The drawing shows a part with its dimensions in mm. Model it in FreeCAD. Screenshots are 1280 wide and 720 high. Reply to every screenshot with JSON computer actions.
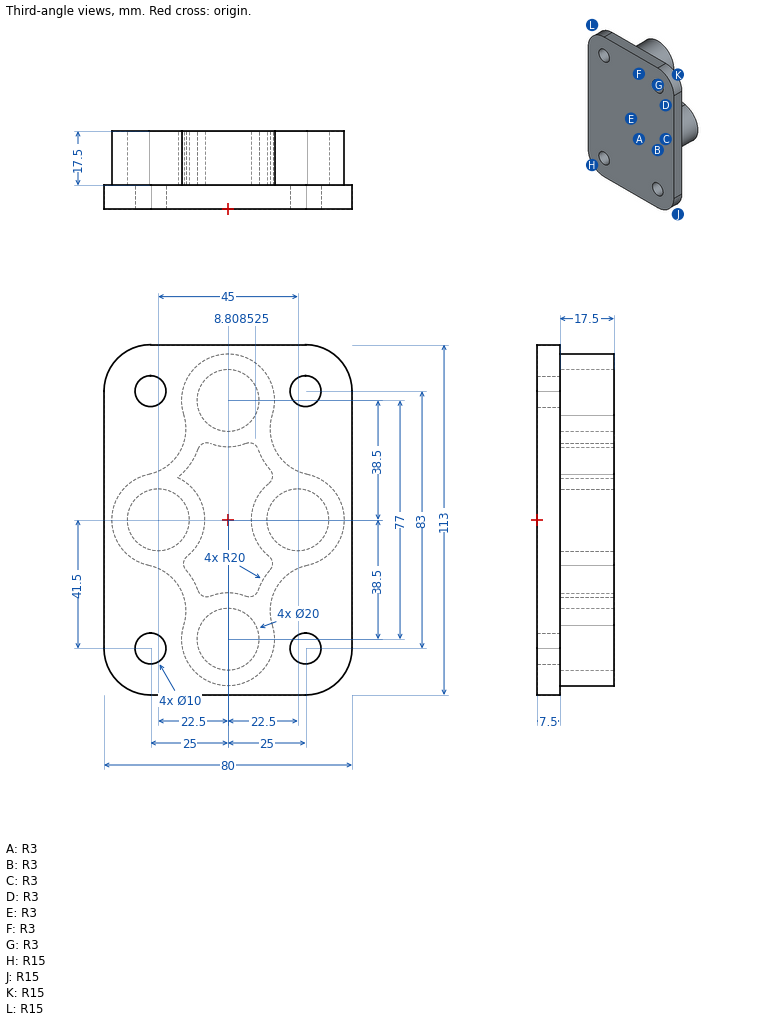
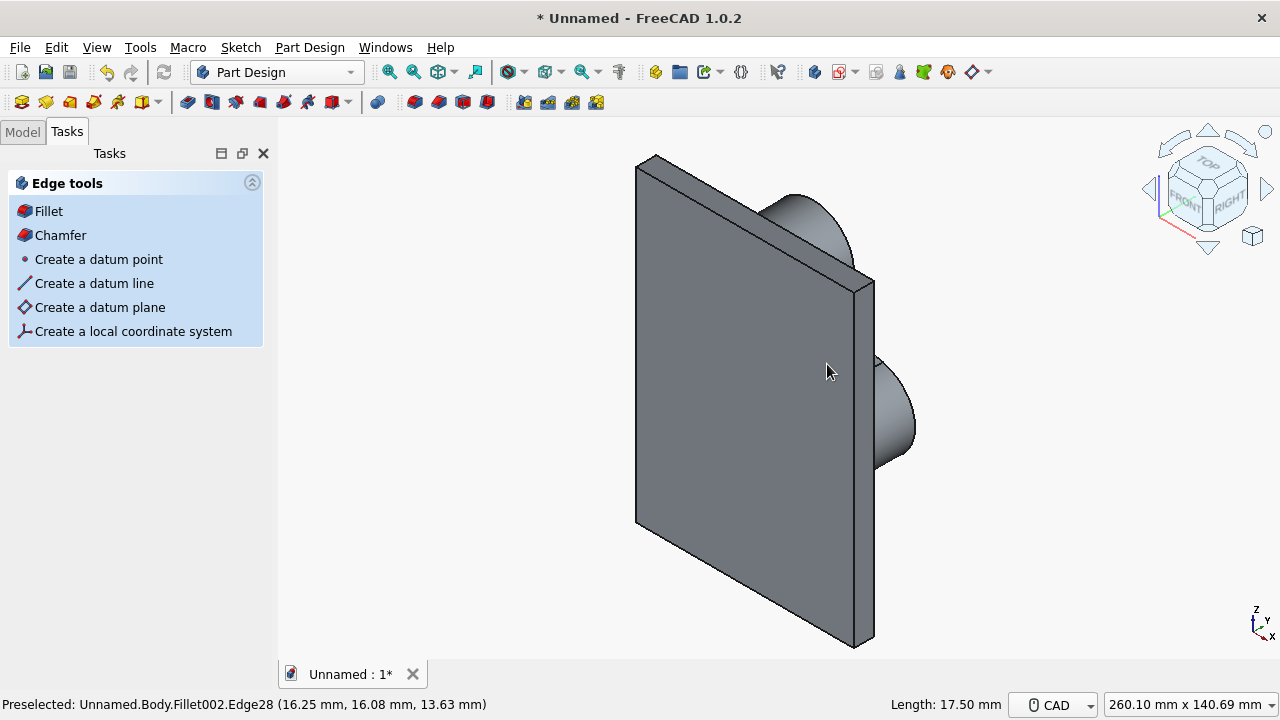
{"action": "left_click", "coordinate": [416, 102]}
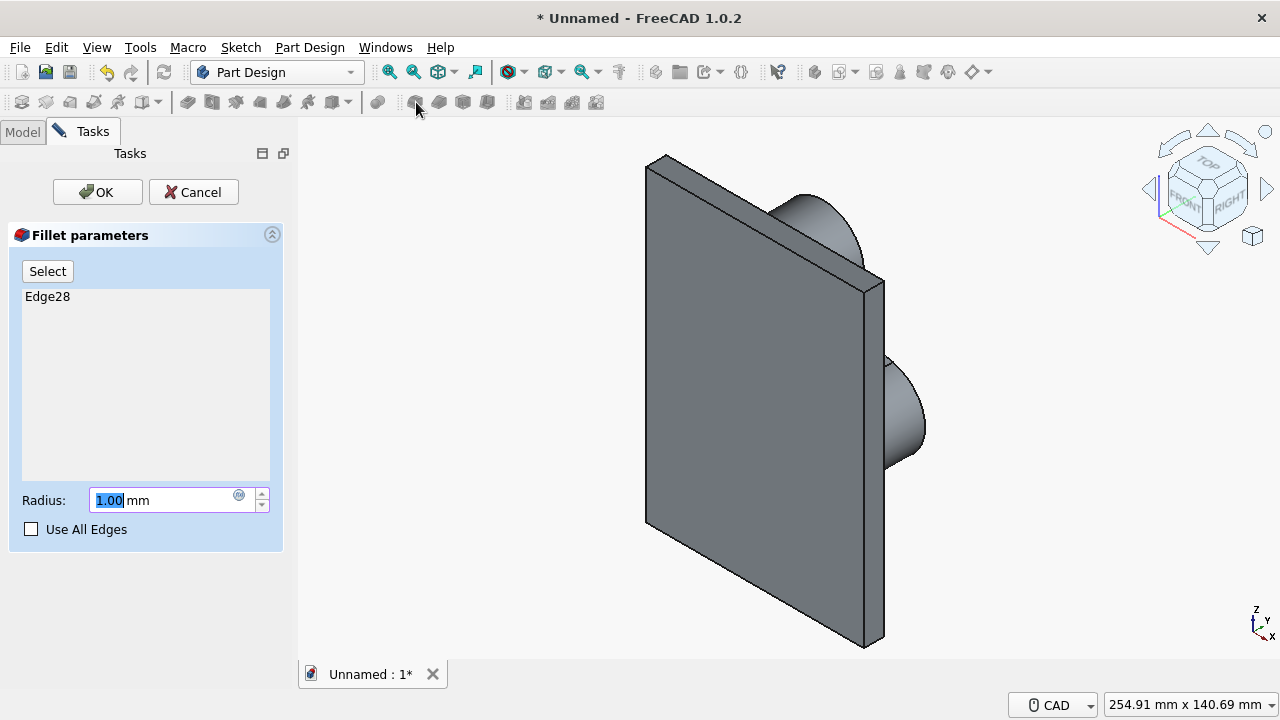
{"action": "type", "text": "3"}
{"action": "key", "text": "Tab"}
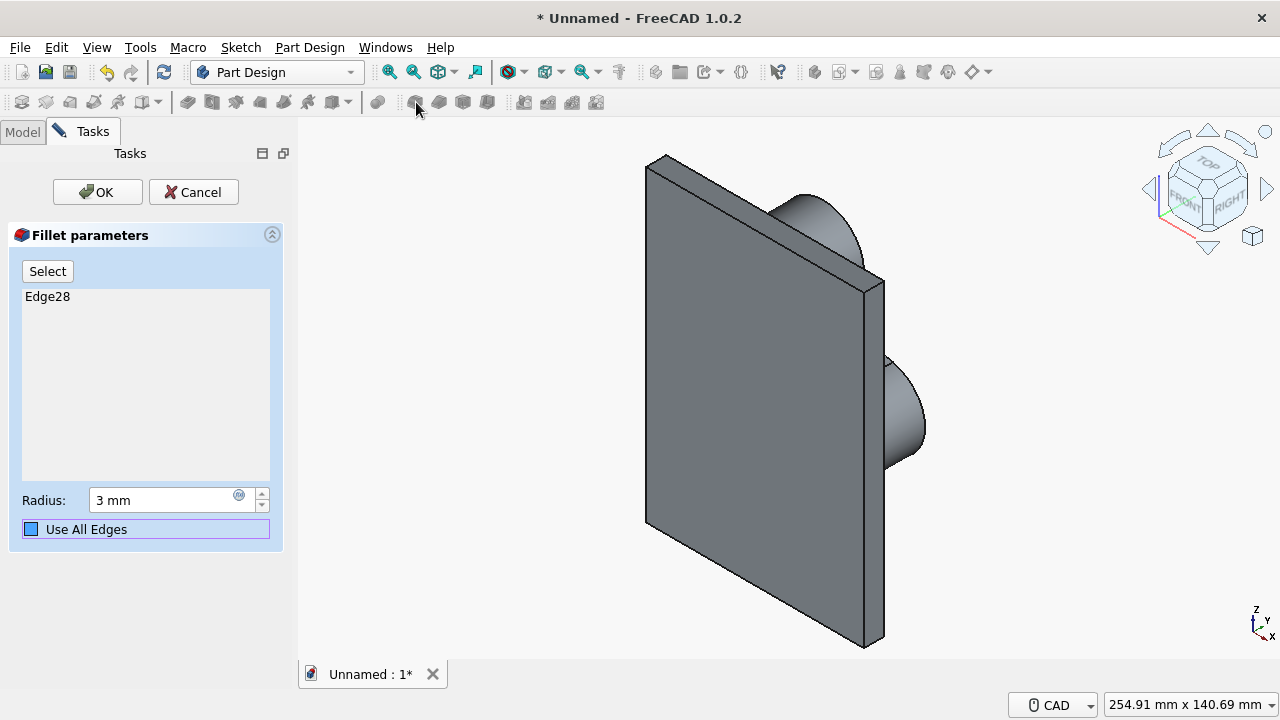
{"action": "left_click", "coordinate": [98, 192]}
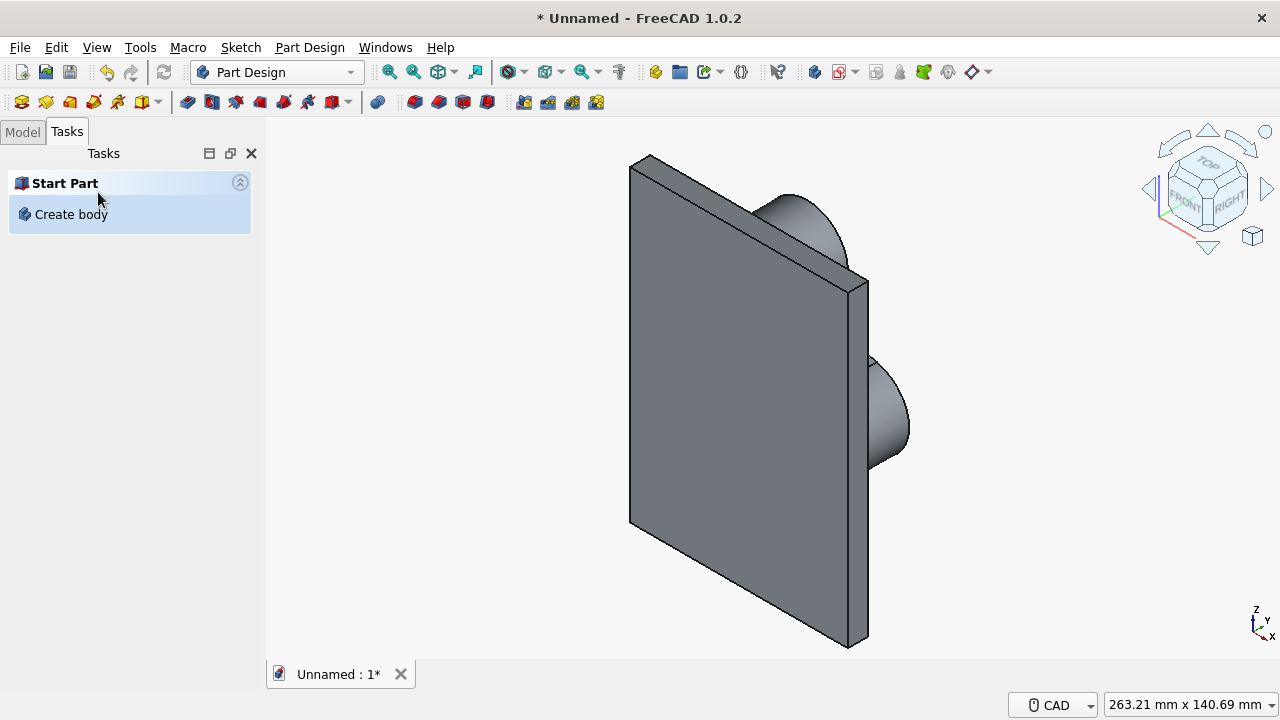
{"action": "key", "text": "2"}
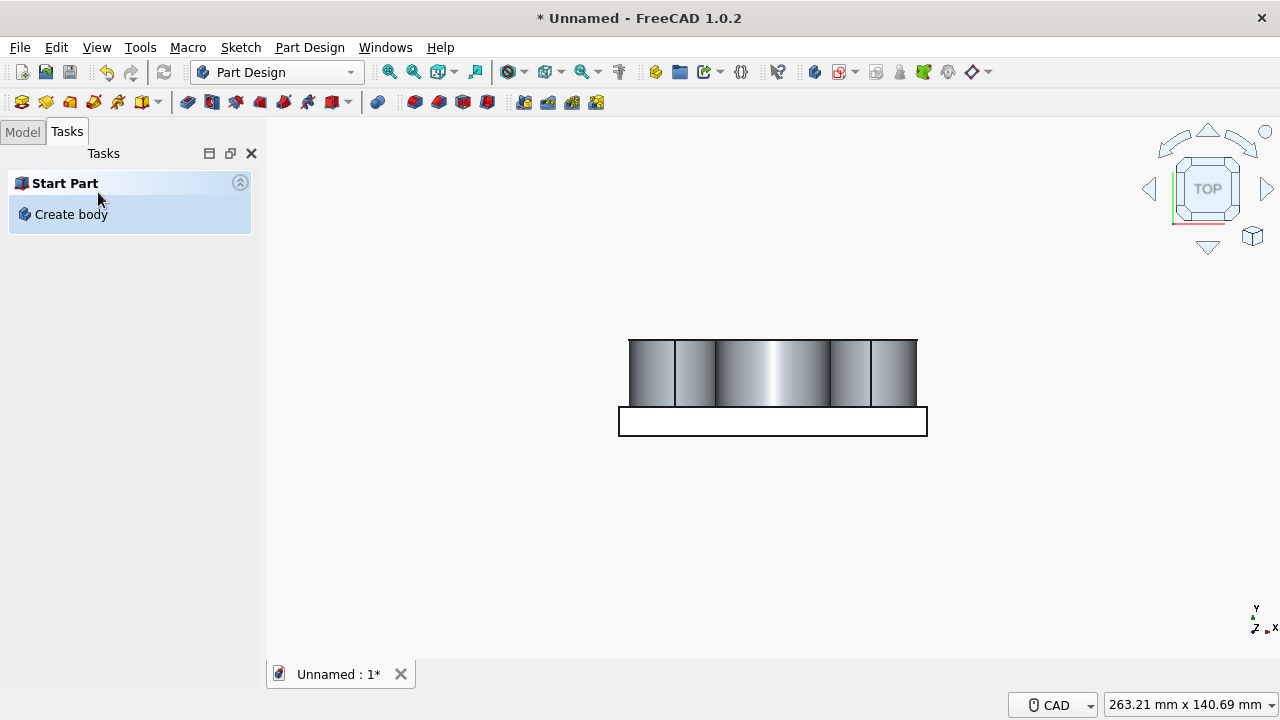
{"action": "key", "text": "v f"}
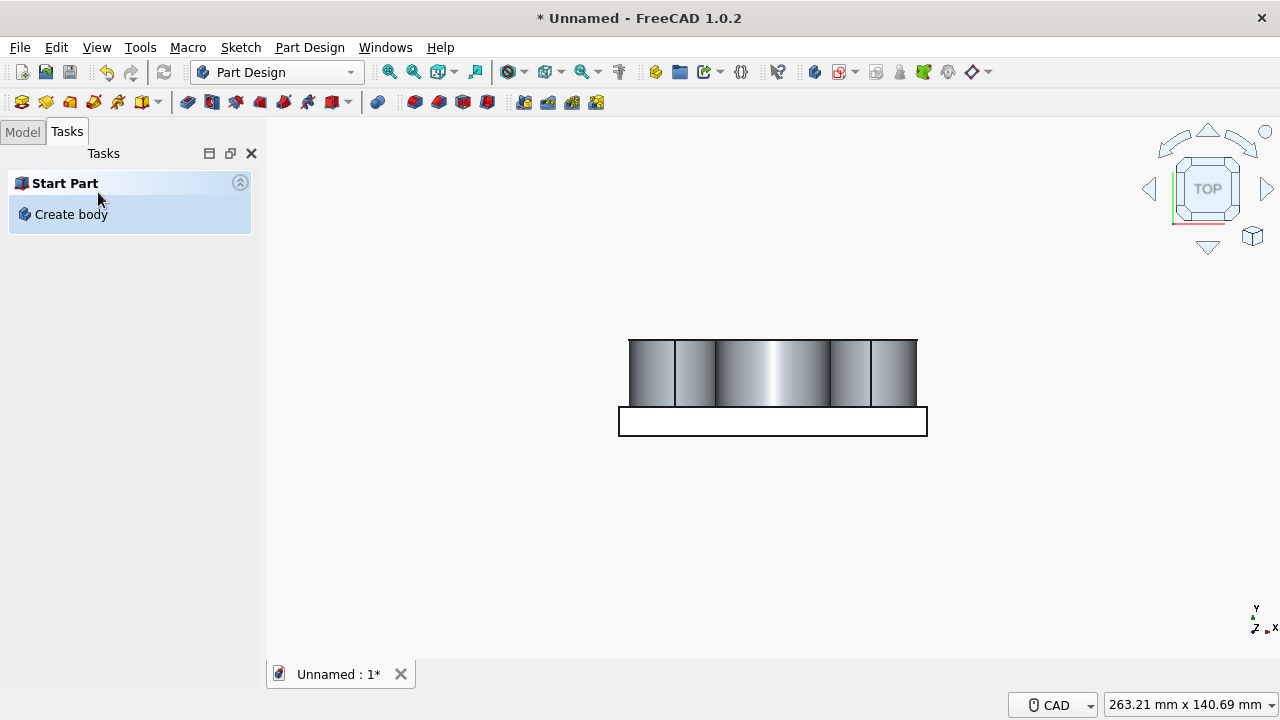
{"action": "key", "text": "0"}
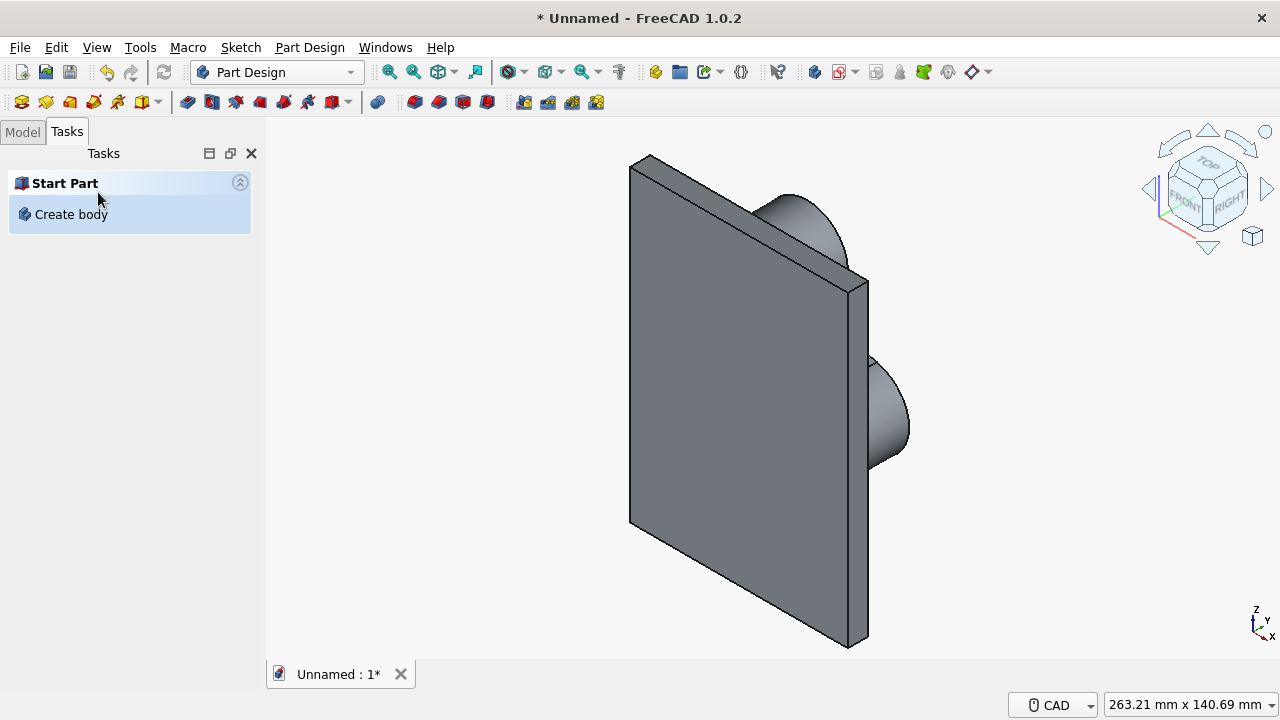
{"action": "key", "text": "1"}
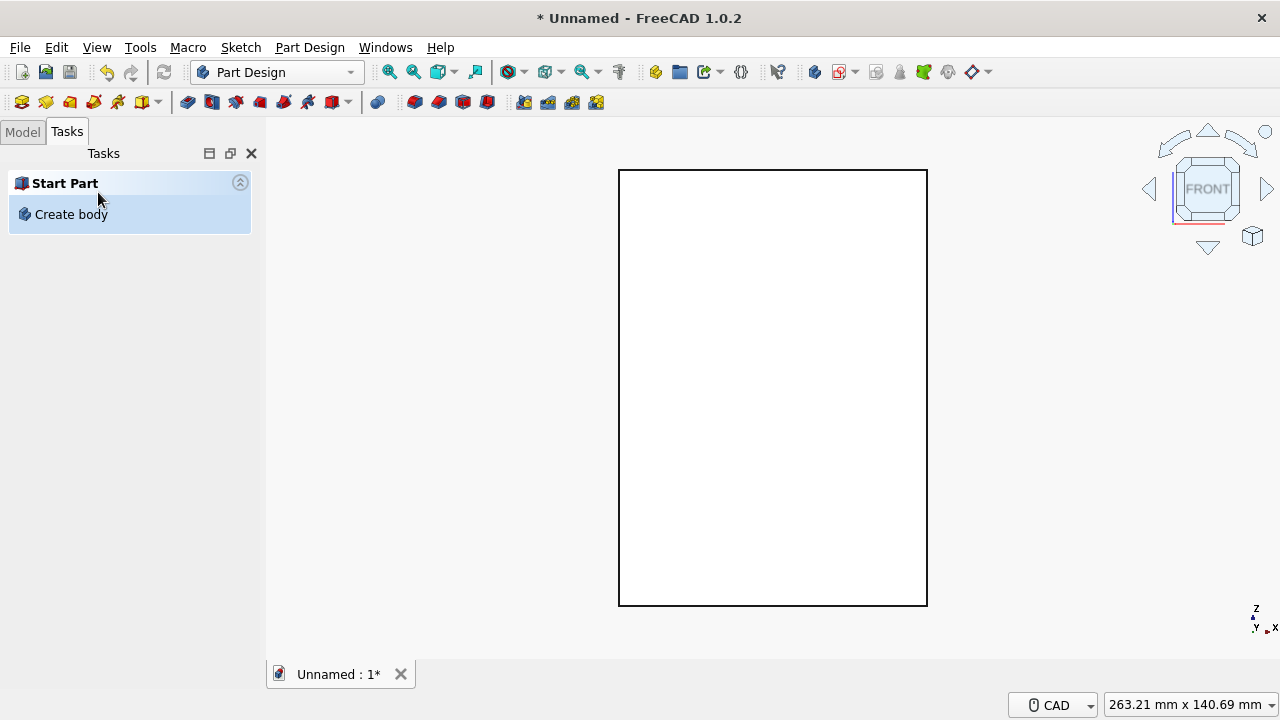
{"action": "key", "text": "3"}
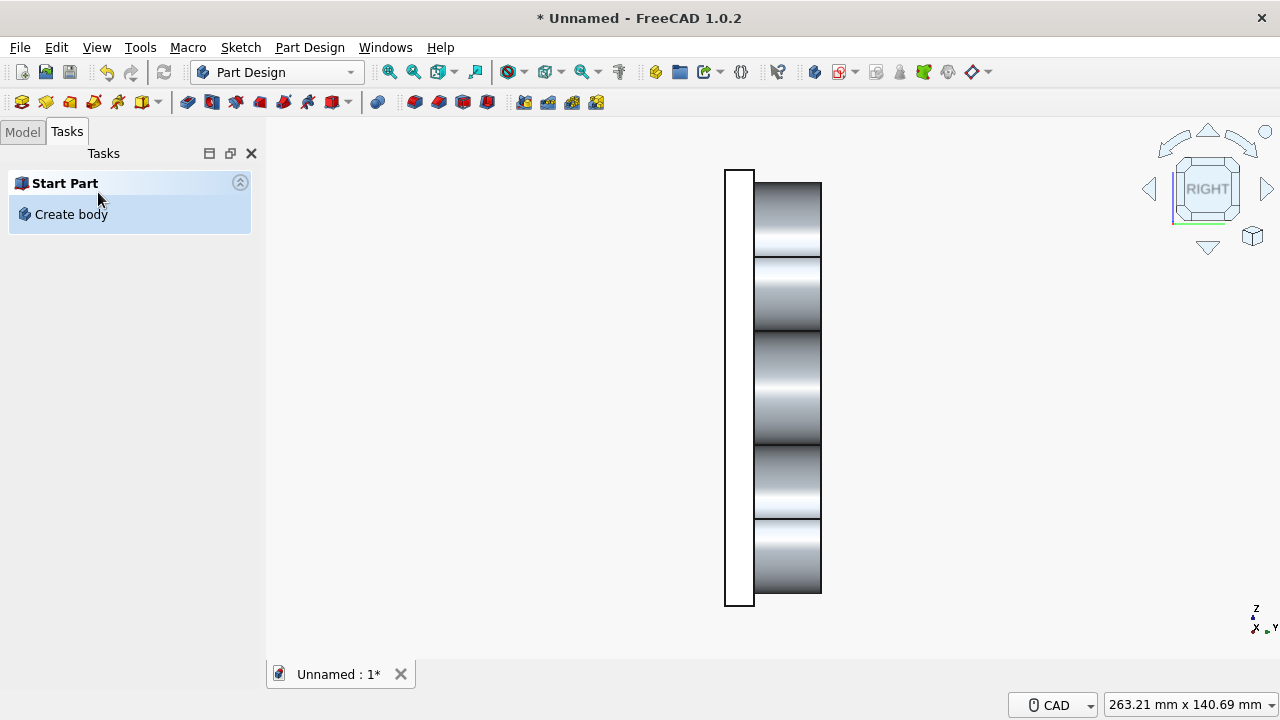
{"action": "key", "text": "5"}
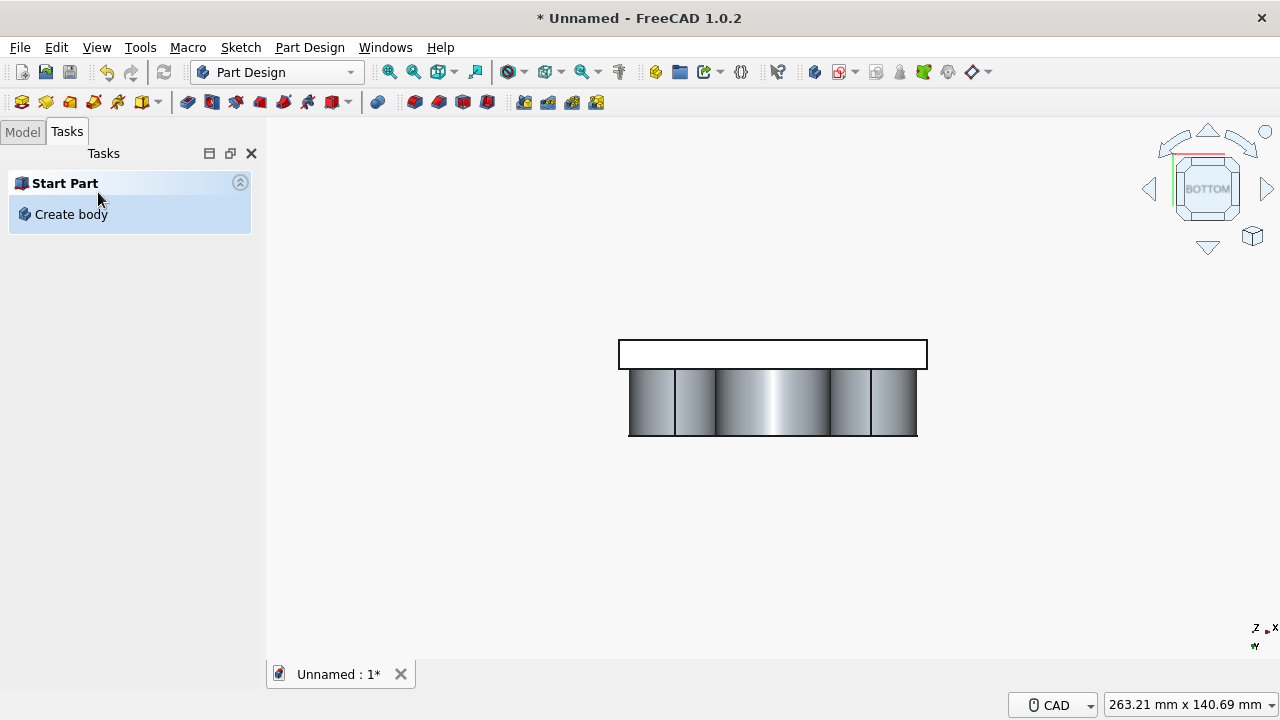
{"action": "left_click", "coordinate": [390, 72]}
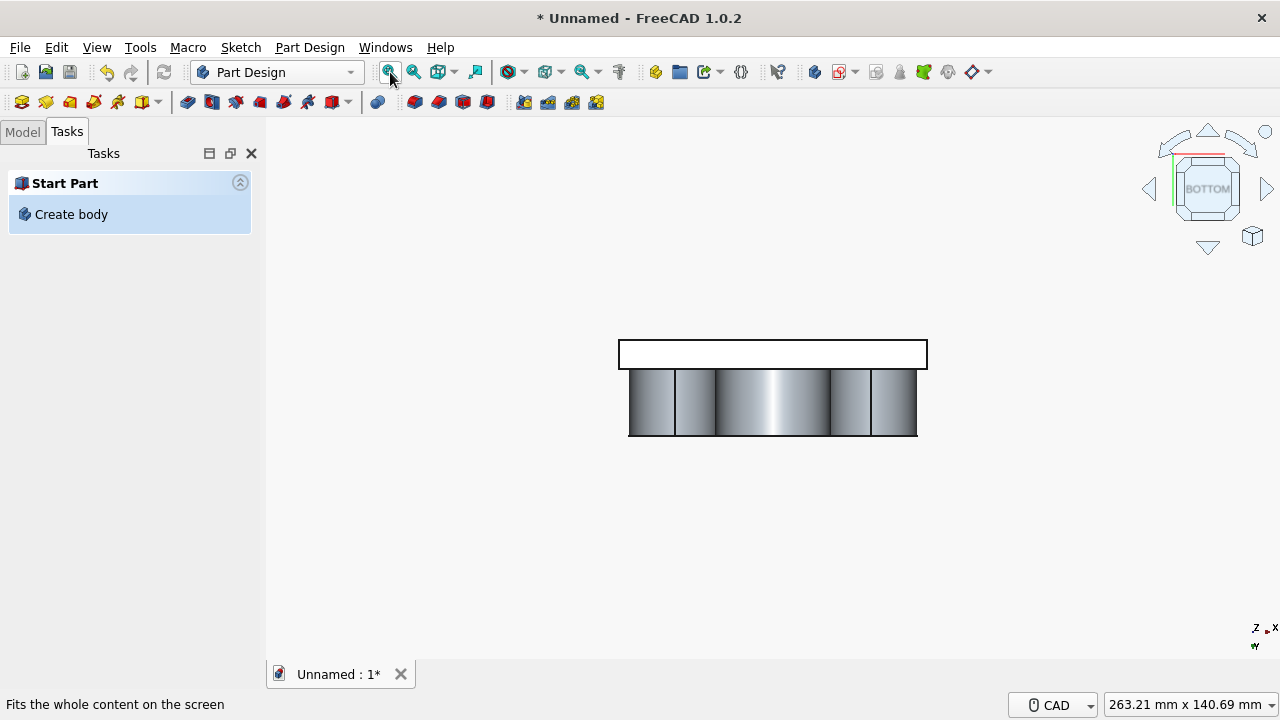
{"action": "key", "text": "4"}